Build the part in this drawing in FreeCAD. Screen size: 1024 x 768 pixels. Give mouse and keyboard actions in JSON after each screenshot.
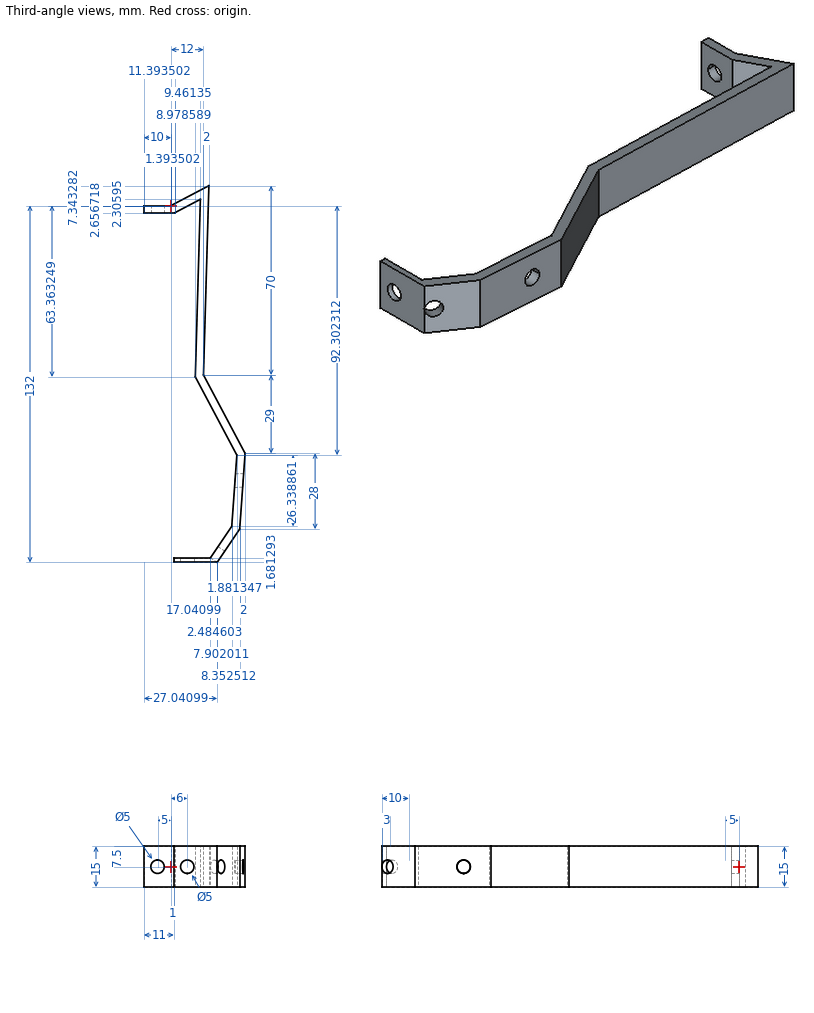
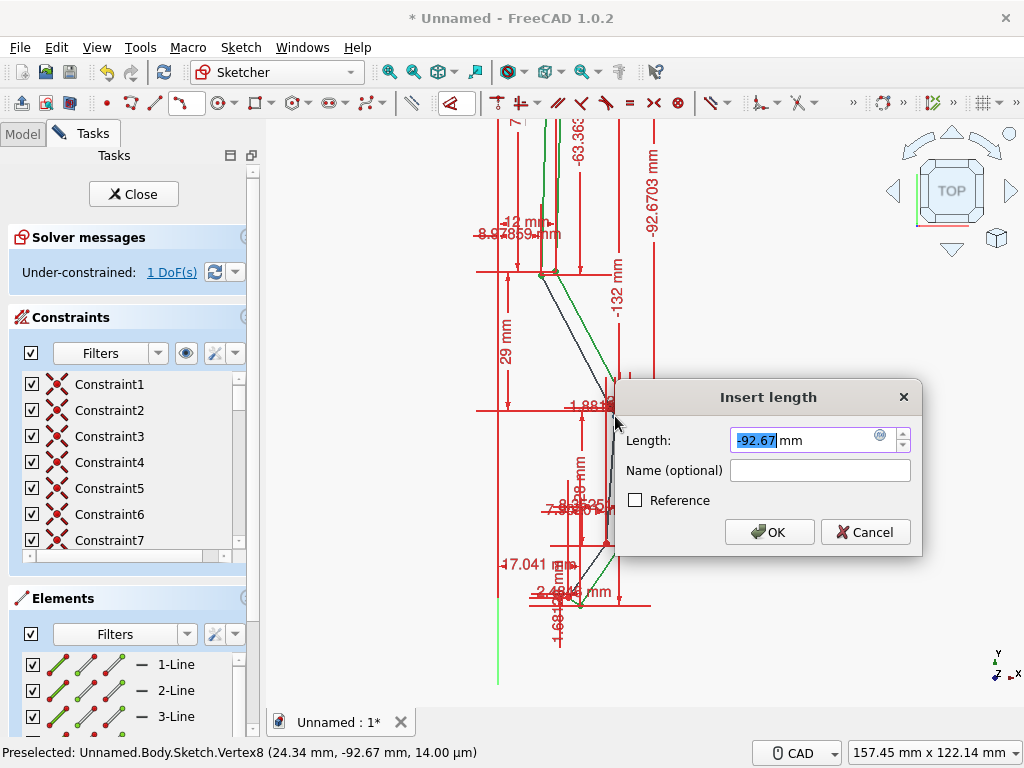
{"action": "type", "text": "-92.302312"}
{"action": "key", "text": "Return"}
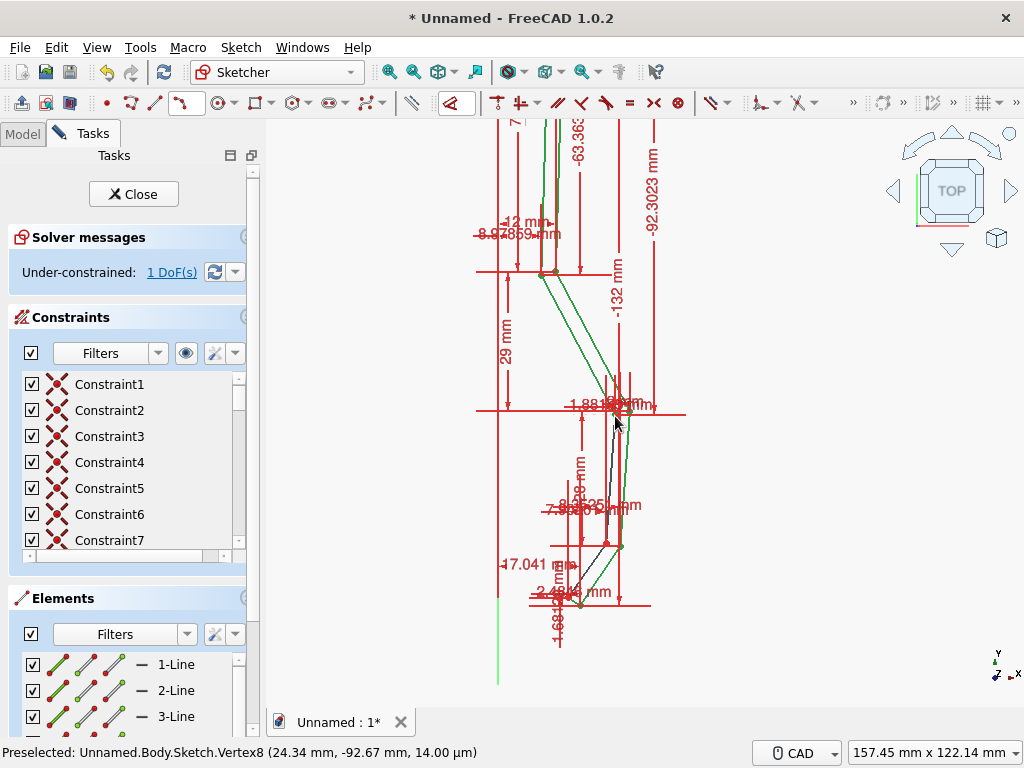
{"action": "left_click", "coordinate": [612, 453]}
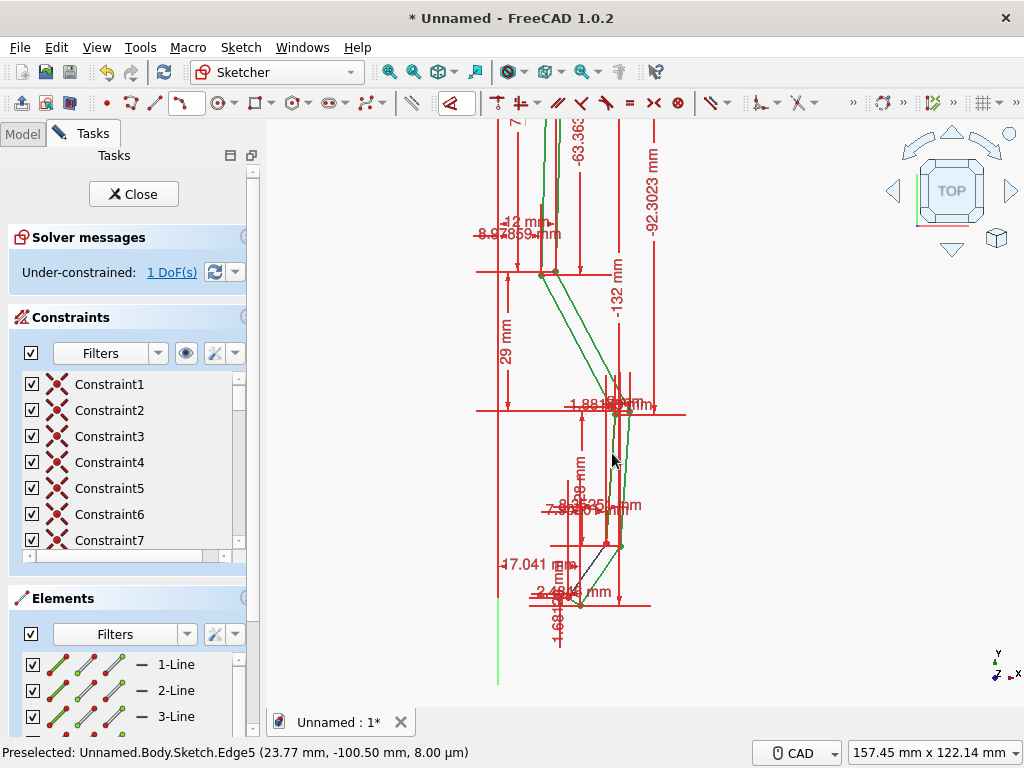
{"action": "left_click", "coordinate": [470, 104]}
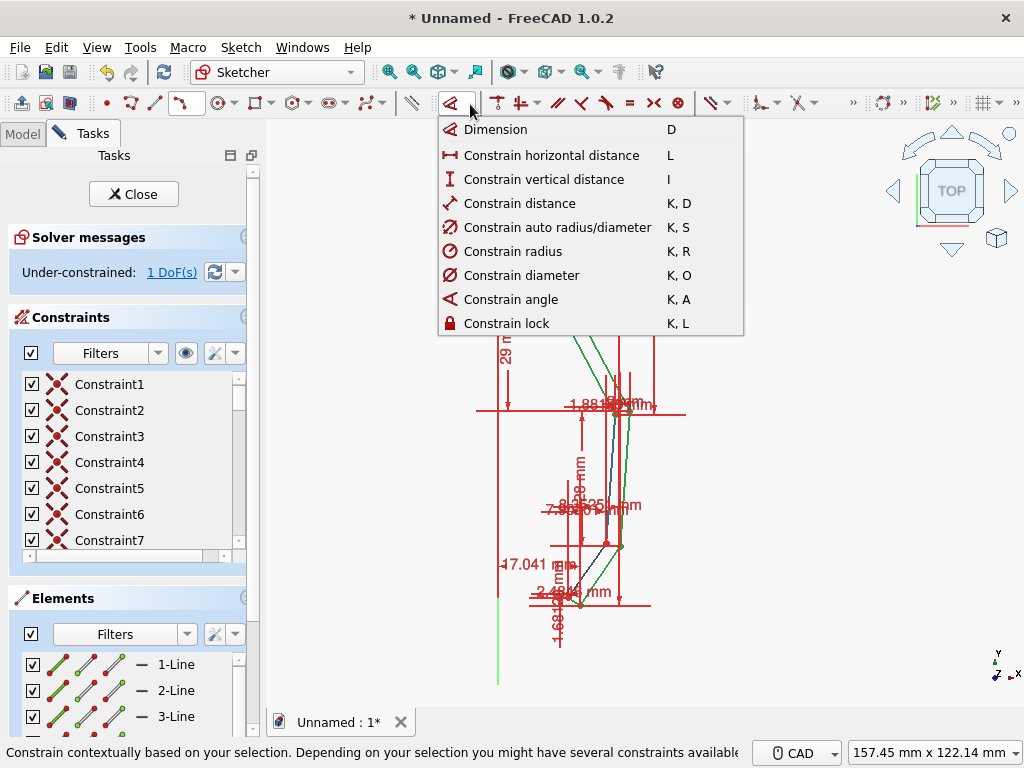
{"action": "left_click", "coordinate": [591, 179]}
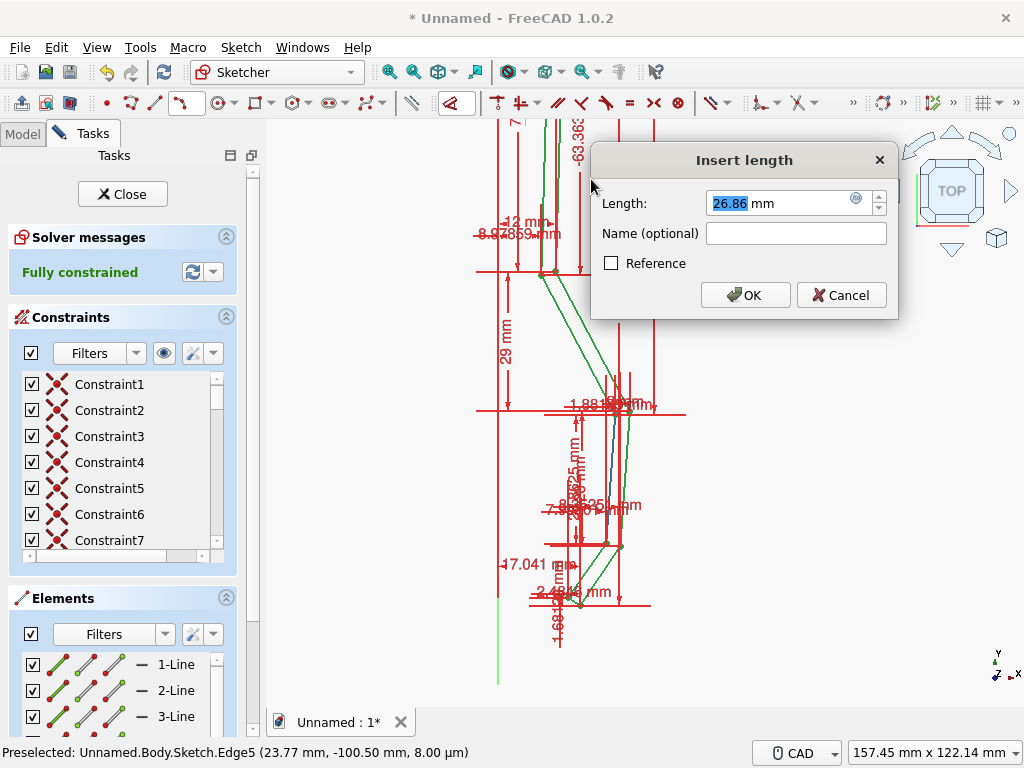
{"action": "type", "text": "26.338861"}
{"action": "key", "text": "Return"}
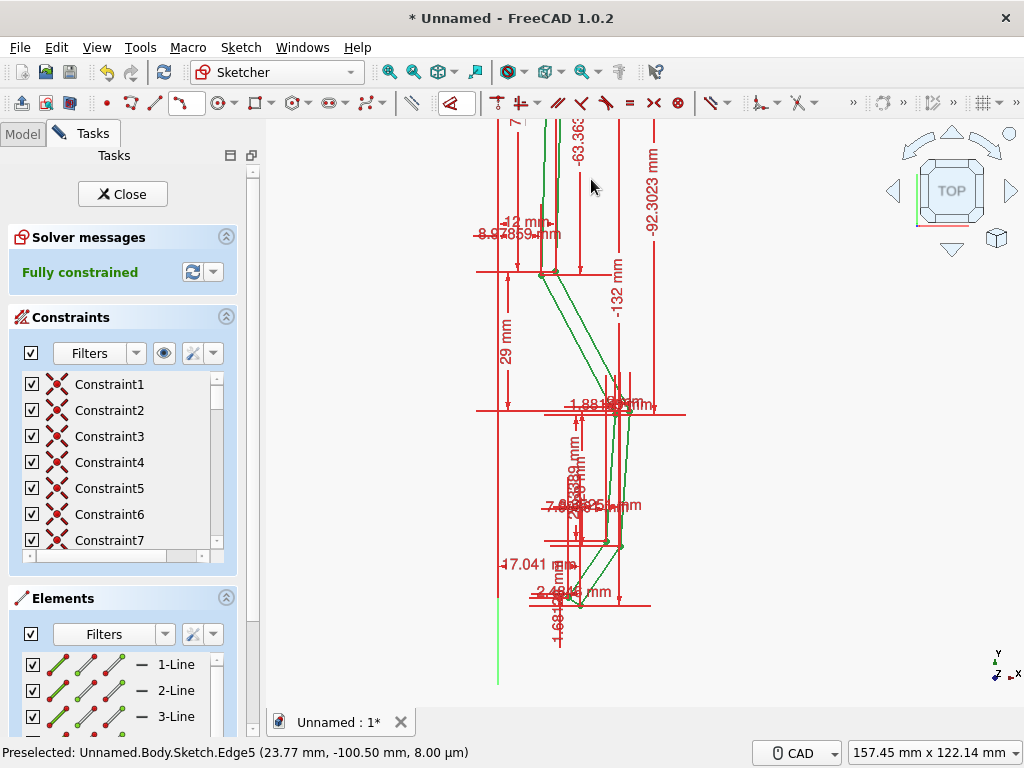
{"action": "left_click", "coordinate": [123, 194]}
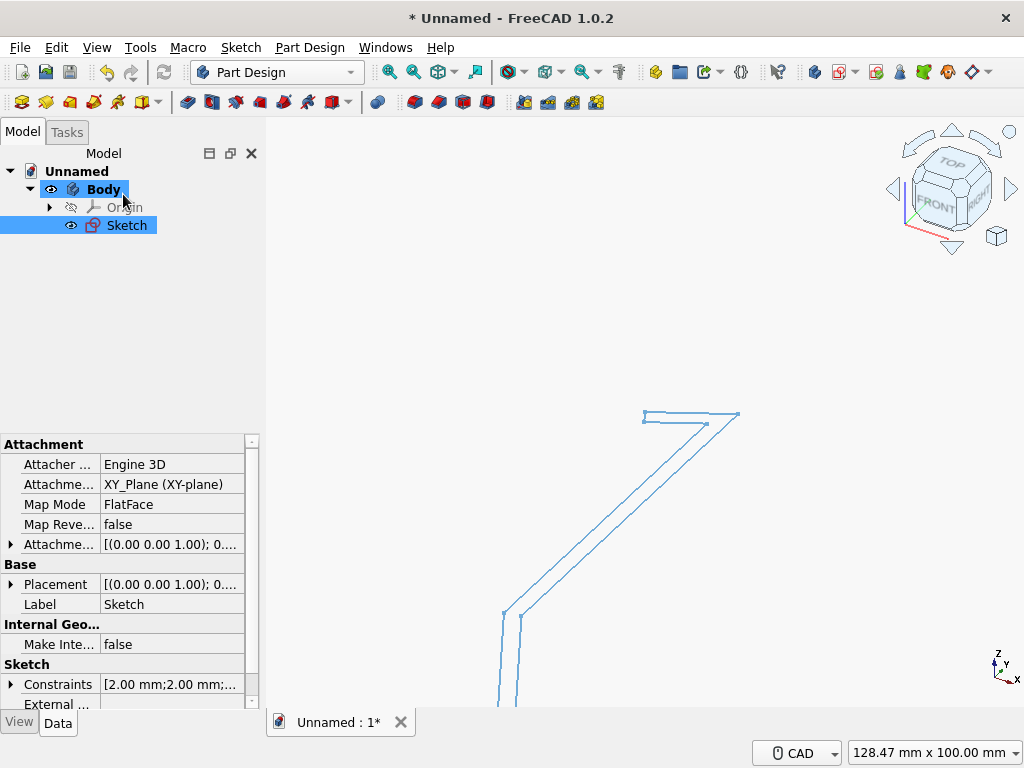
{"action": "left_click", "coordinate": [22, 102]}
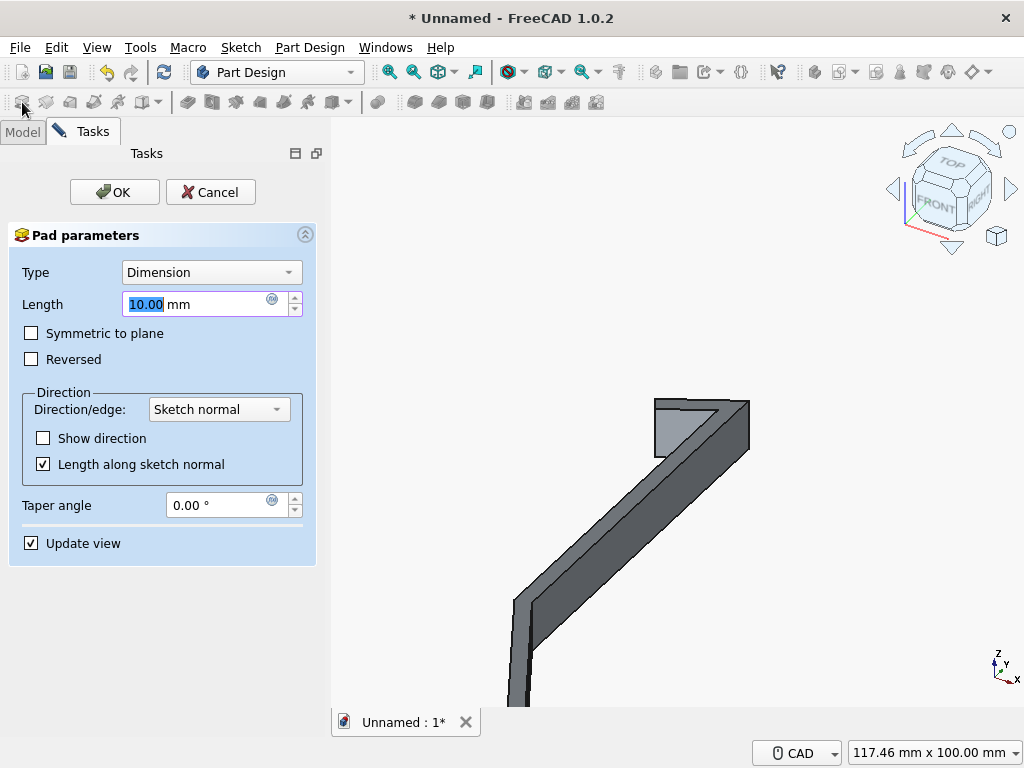
{"action": "type", "text": "15"}
{"action": "key", "text": "Tab"}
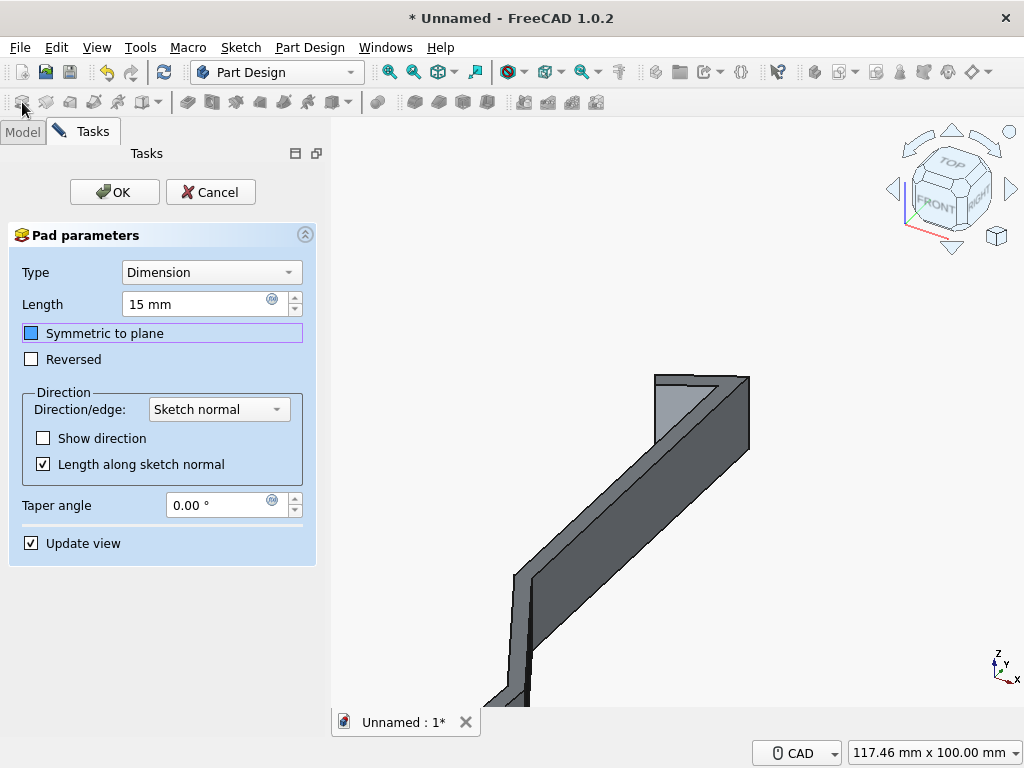
{"action": "left_click", "coordinate": [30, 333]}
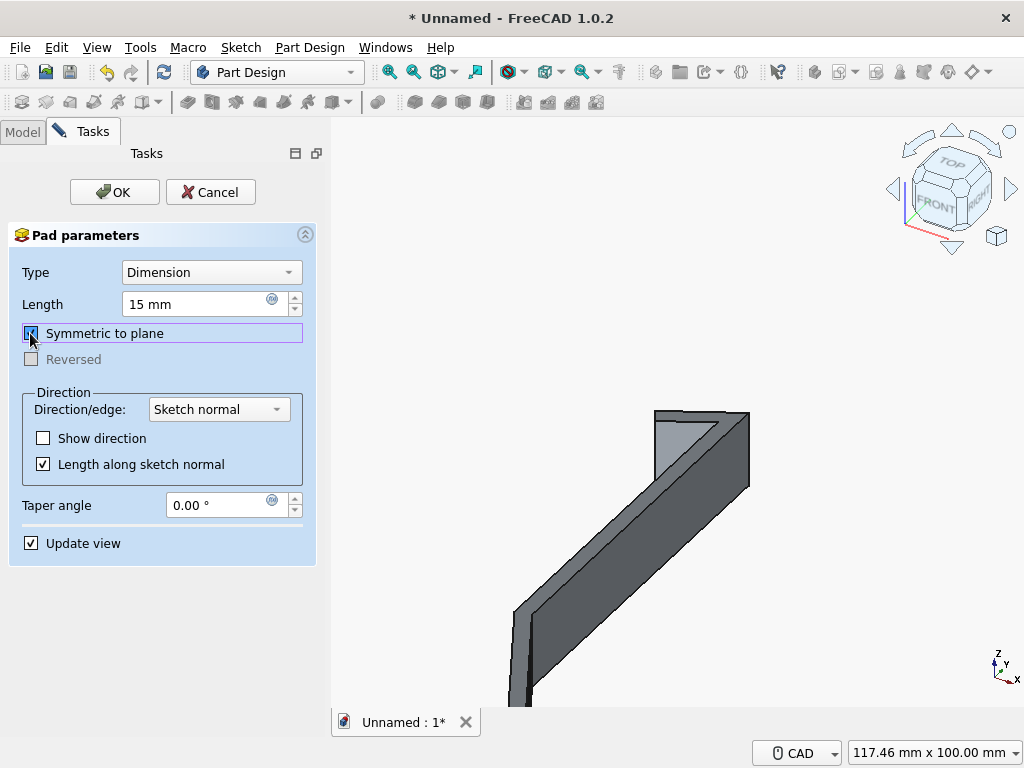
{"action": "left_click", "coordinate": [115, 192]}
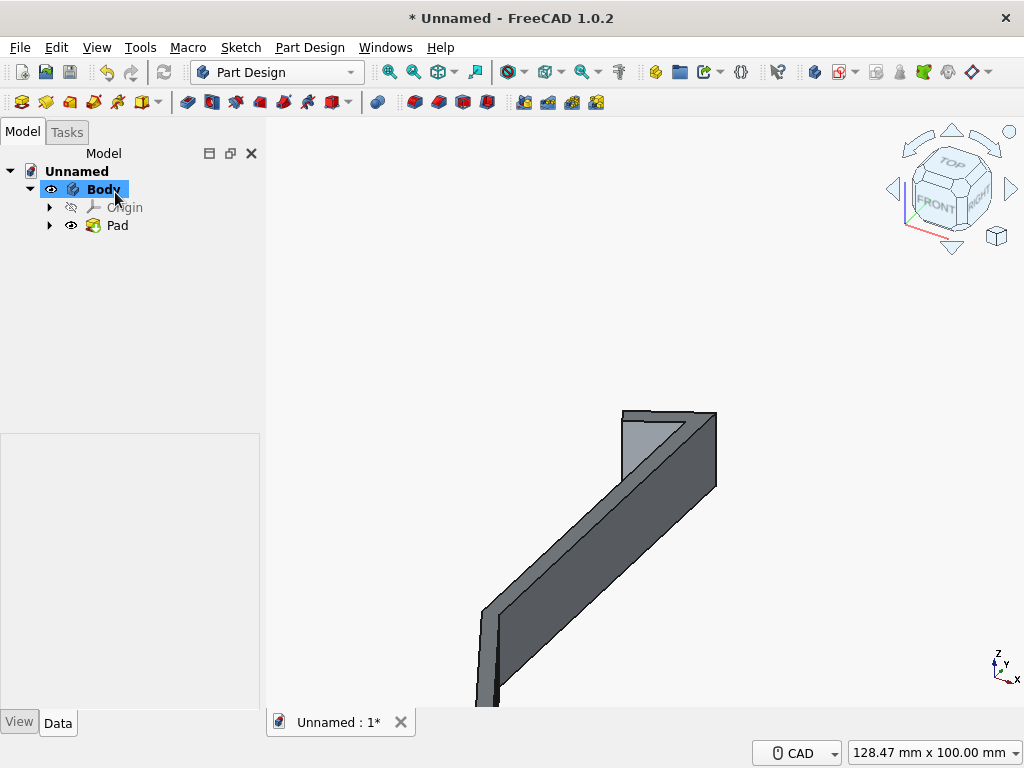
{"action": "left_click", "coordinate": [390, 72]}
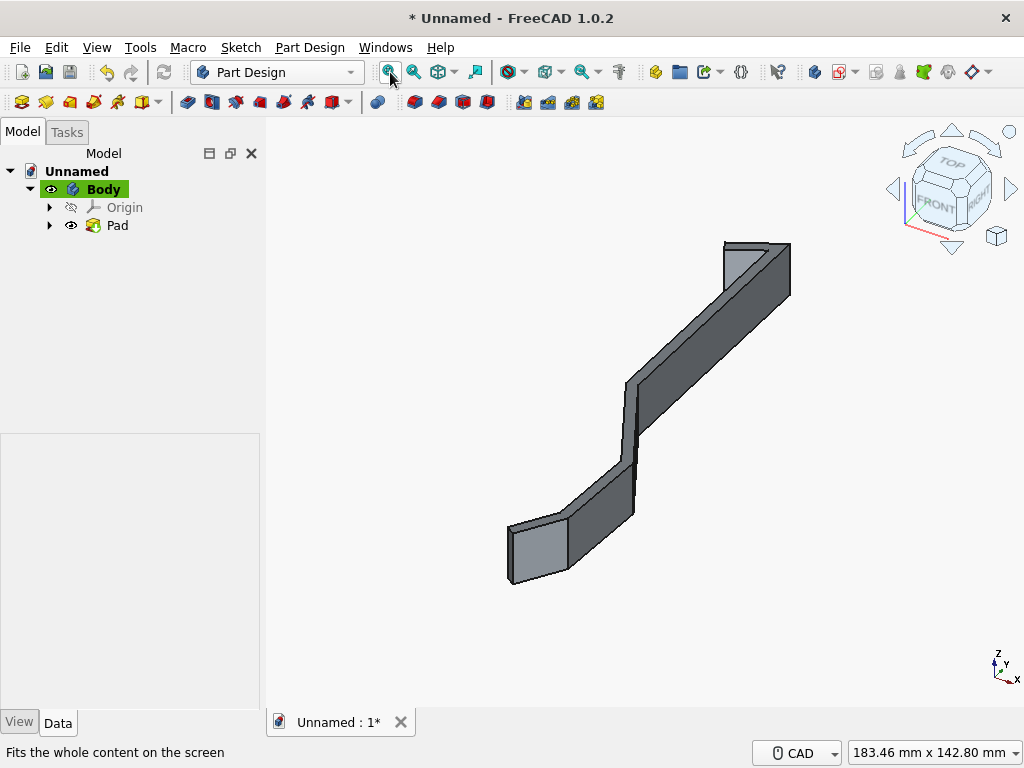
{"action": "scroll", "coordinate": [605, 481], "scroll_direction": "up", "scroll_amount": 5}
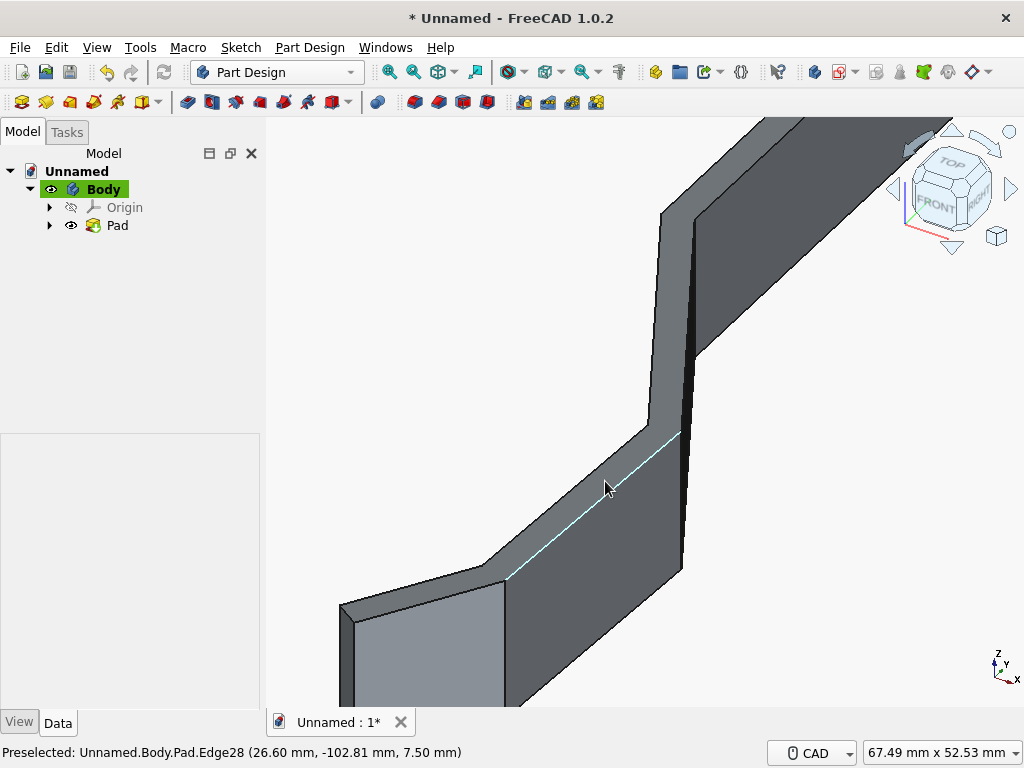
{"action": "left_click", "coordinate": [604, 482]}